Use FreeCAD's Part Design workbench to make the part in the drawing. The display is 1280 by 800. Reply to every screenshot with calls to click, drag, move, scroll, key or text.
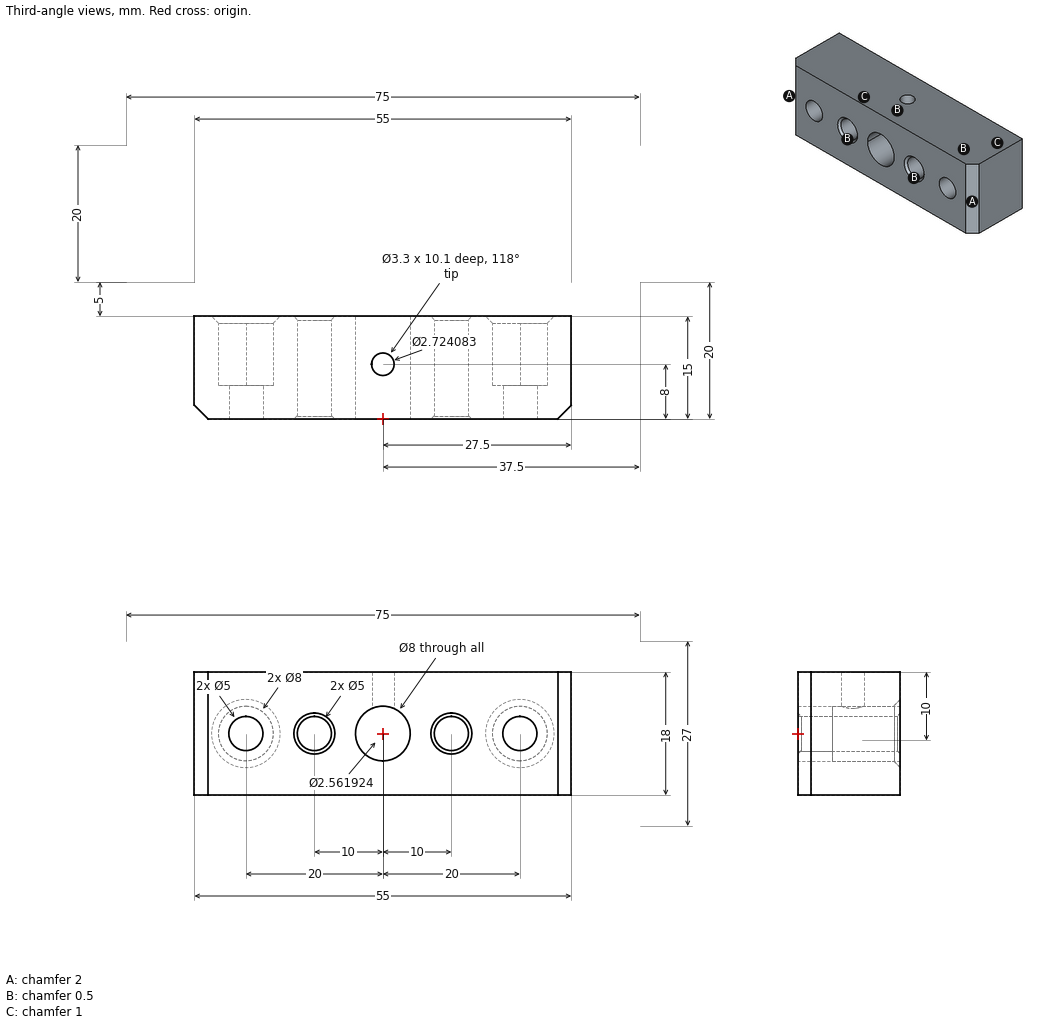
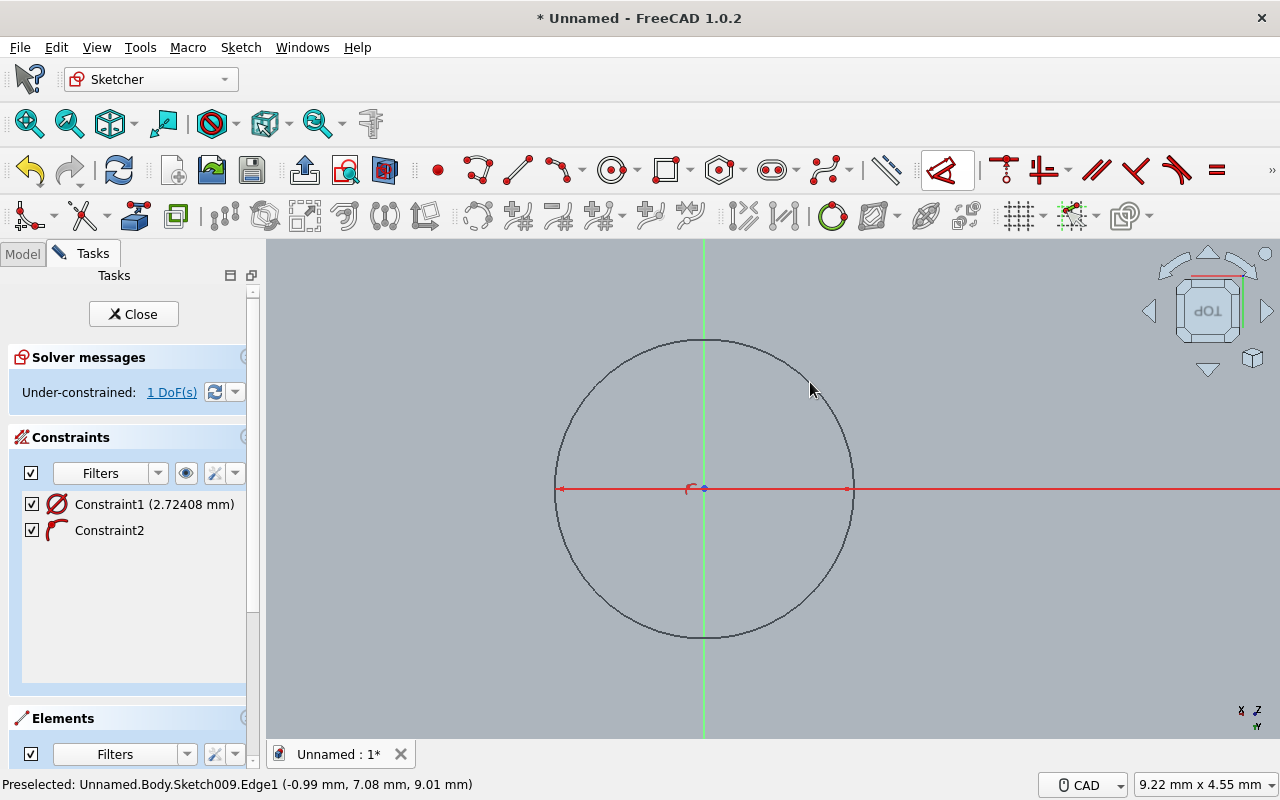
click(704, 489)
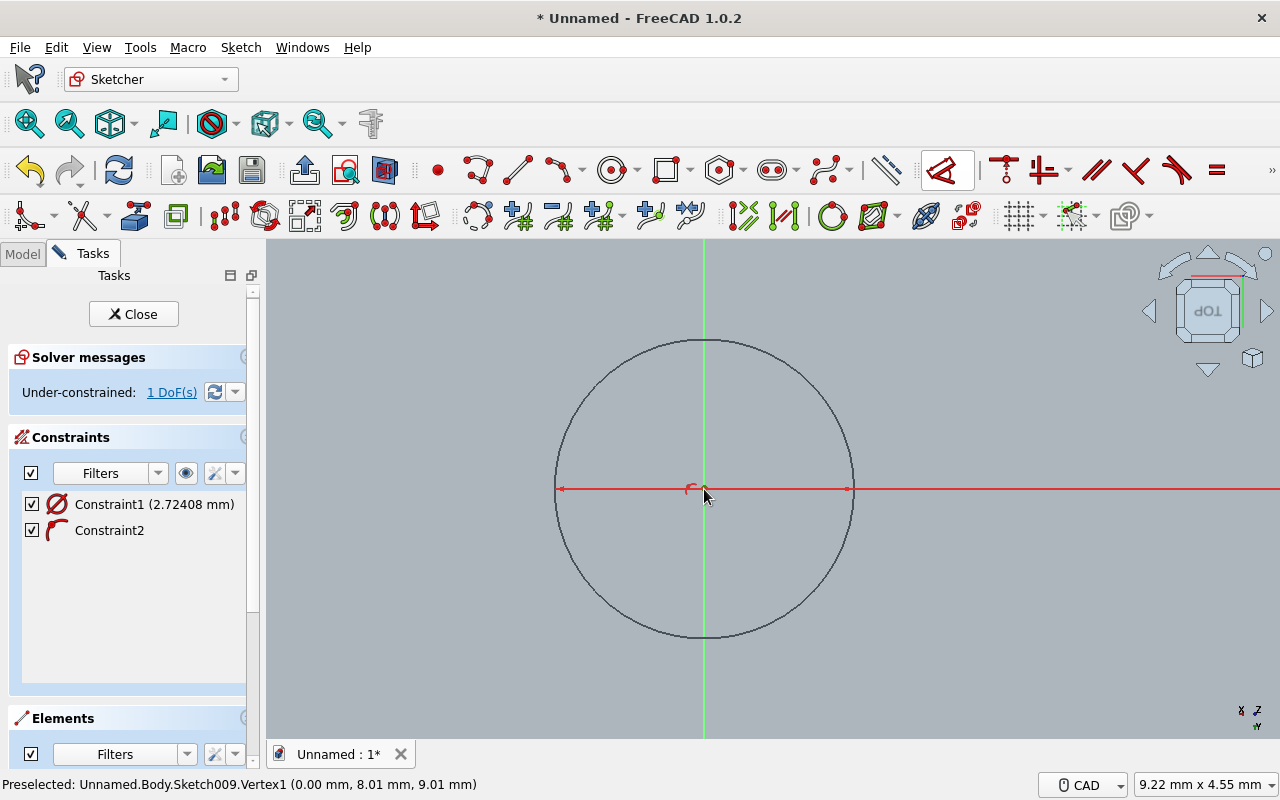
click(968, 170)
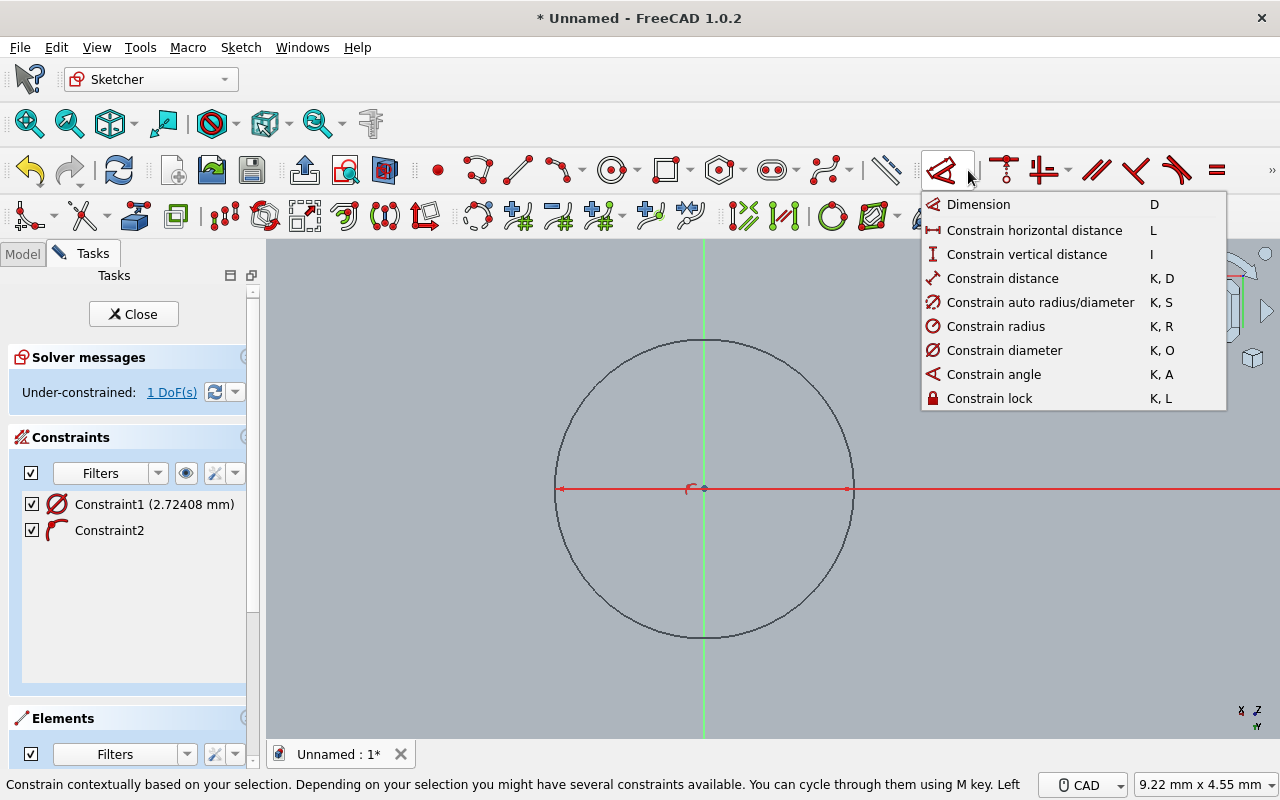
click(1074, 254)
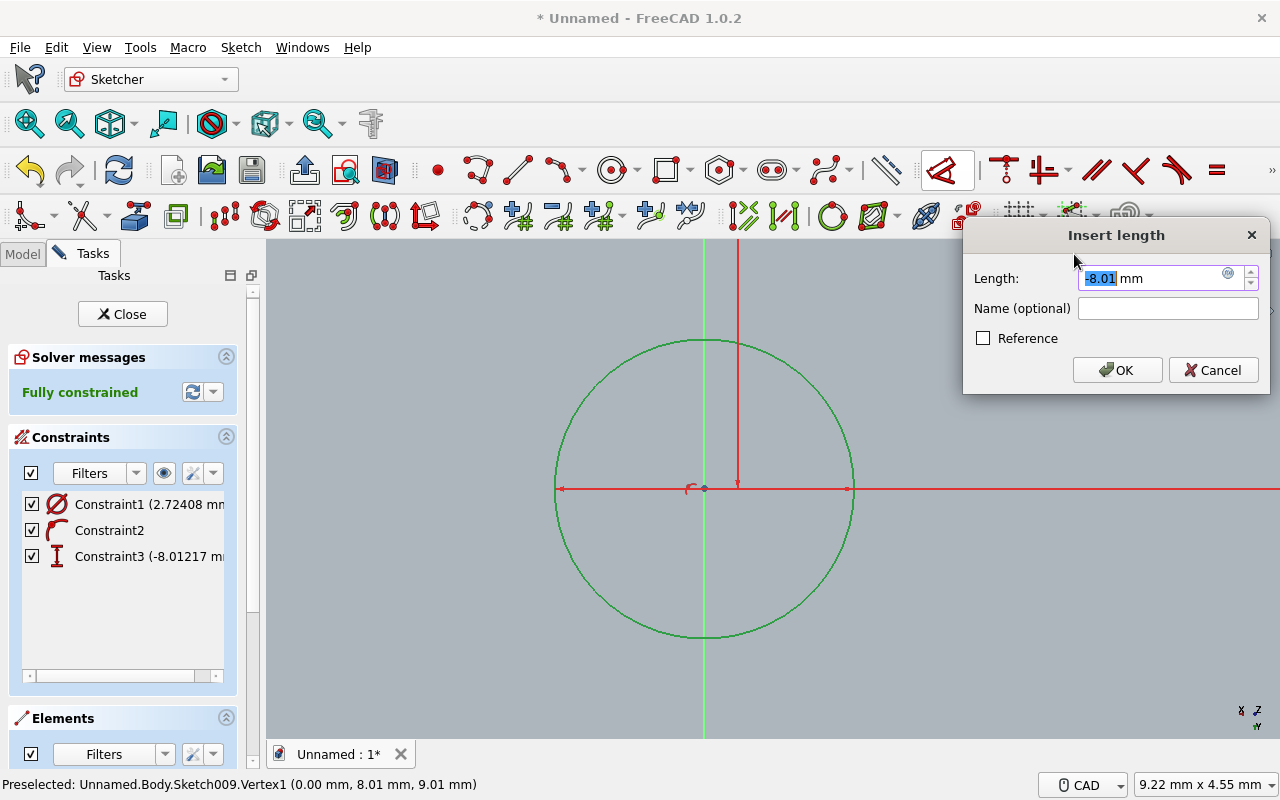
text(-8)
key(Return)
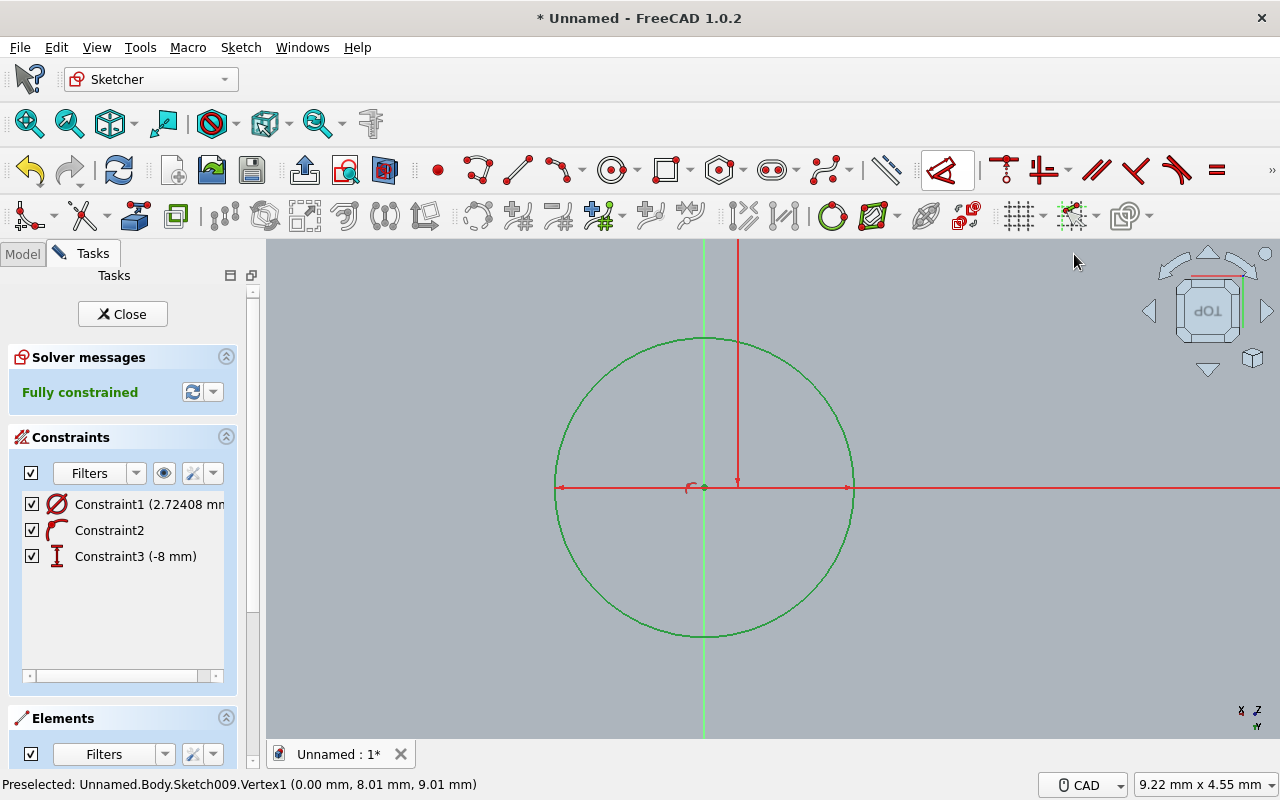
click(123, 314)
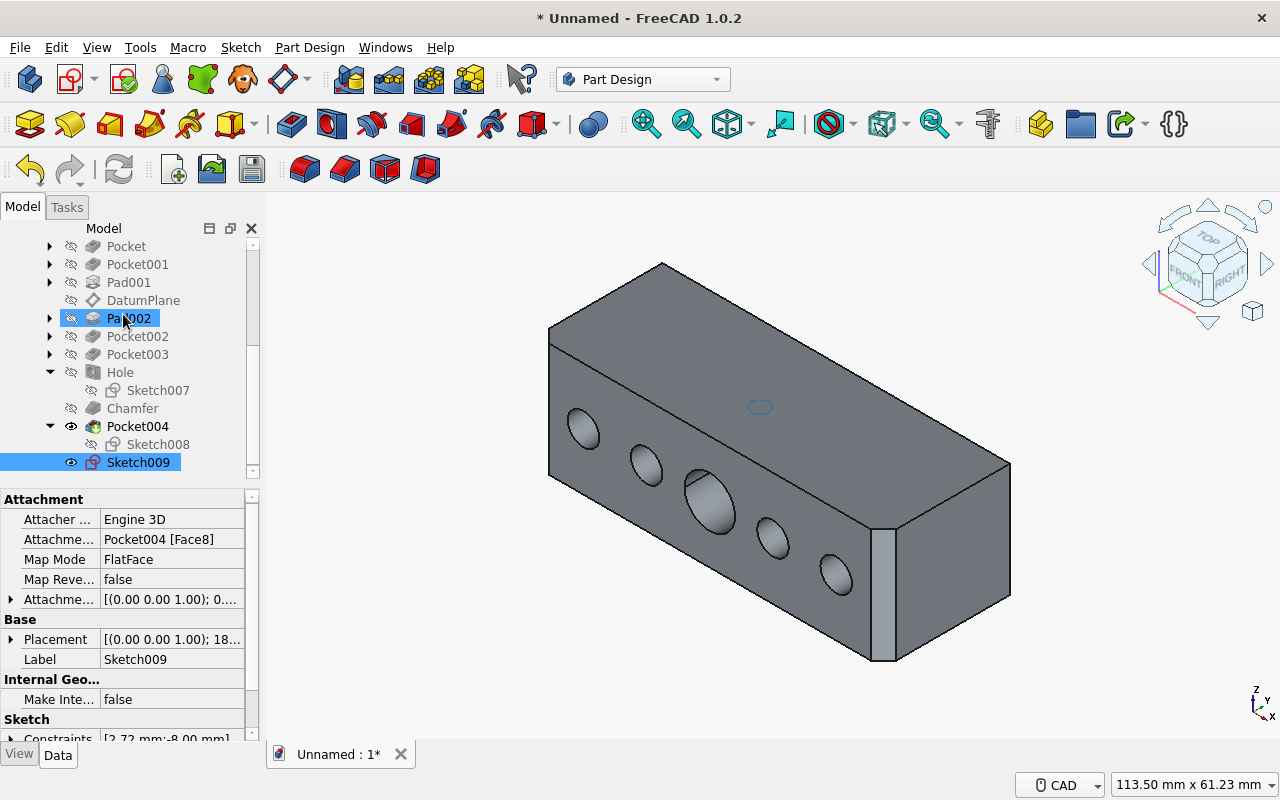
click(292, 124)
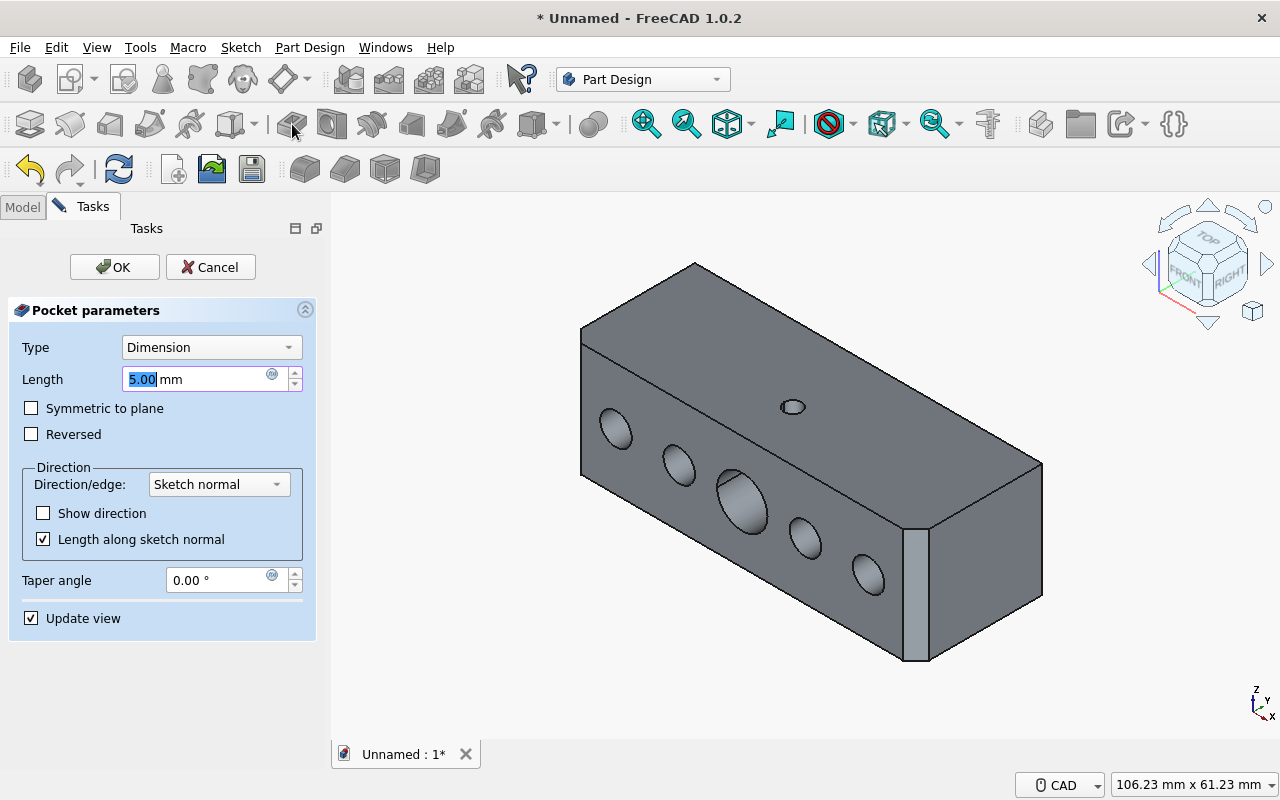
text(10)
key(Tab)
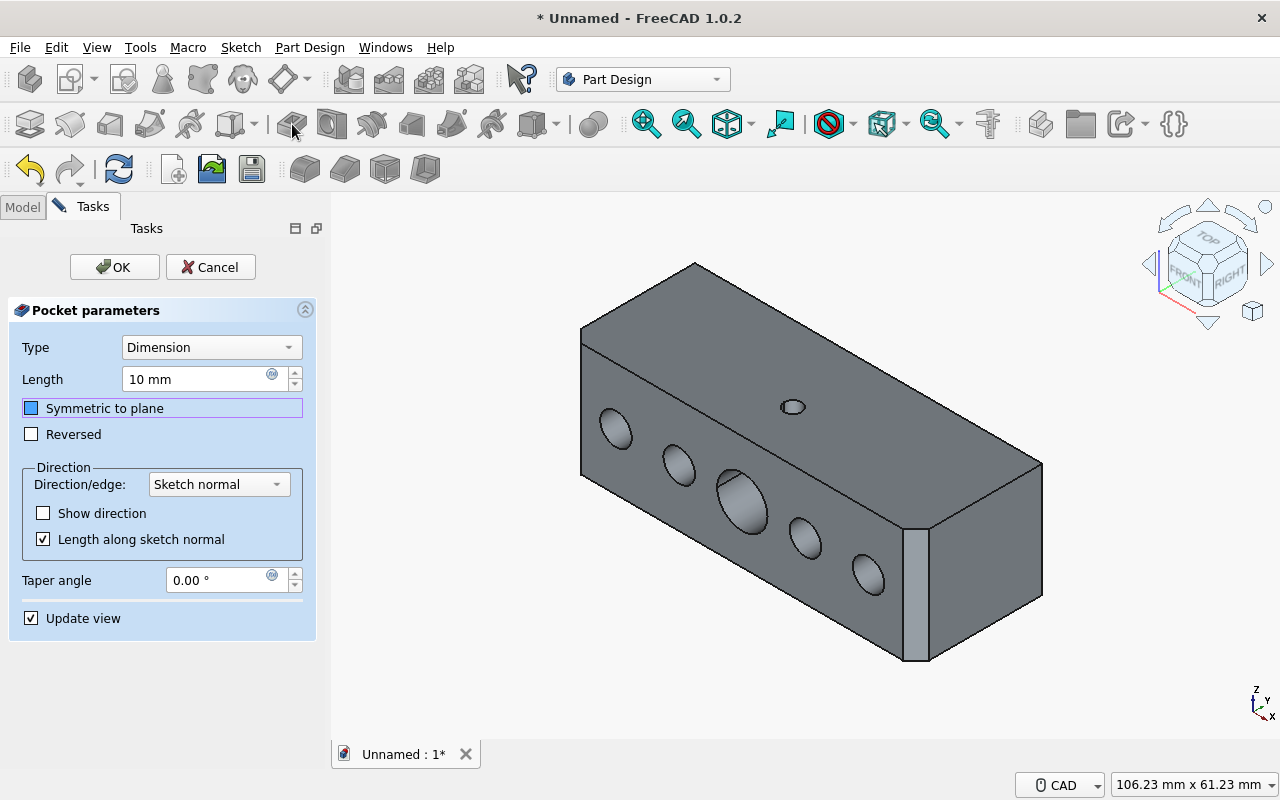
click(115, 267)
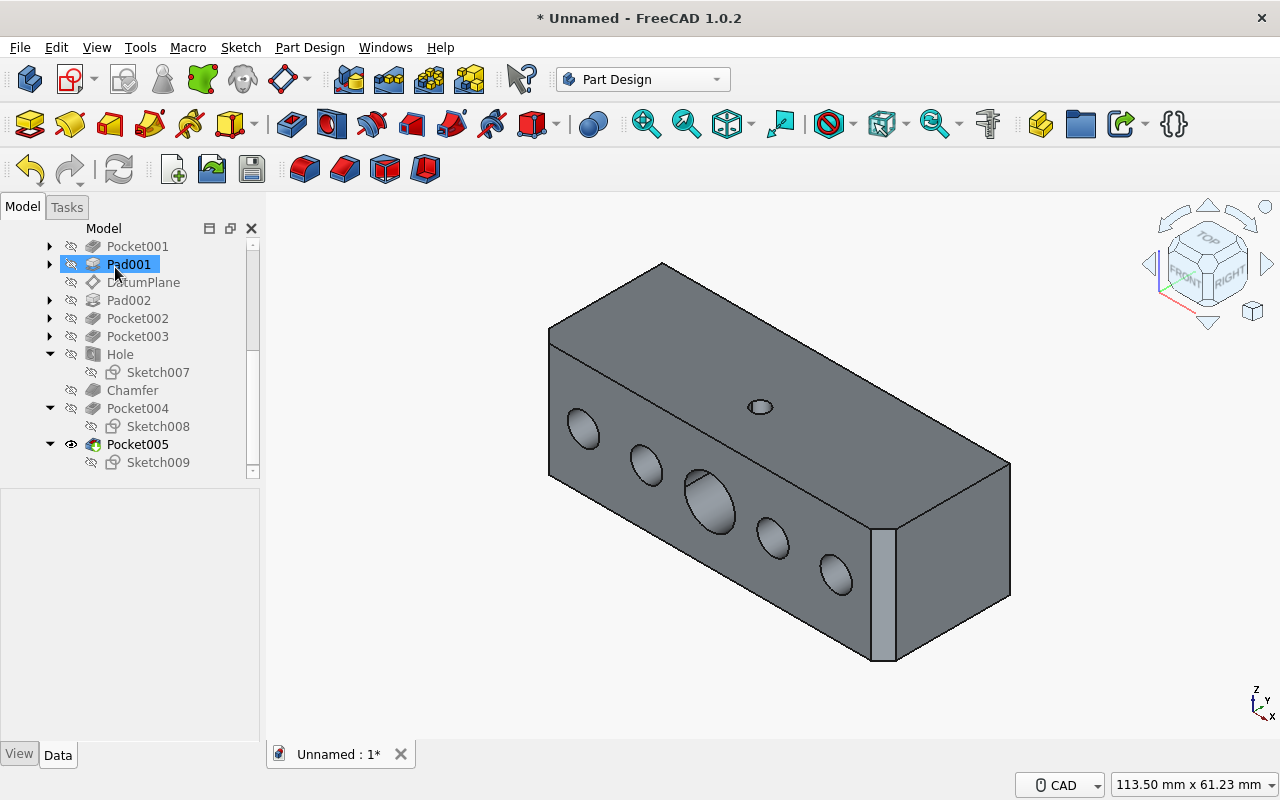
click(872, 456)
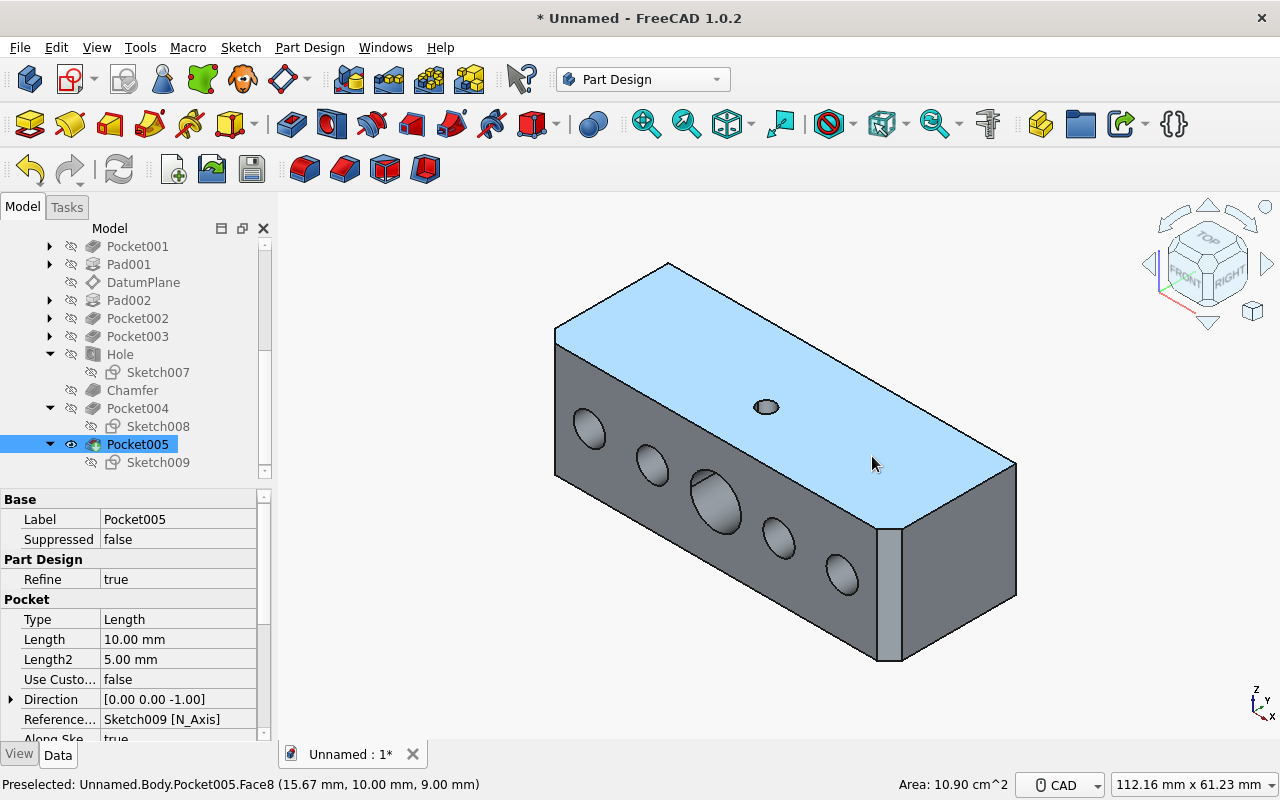
click(70, 80)